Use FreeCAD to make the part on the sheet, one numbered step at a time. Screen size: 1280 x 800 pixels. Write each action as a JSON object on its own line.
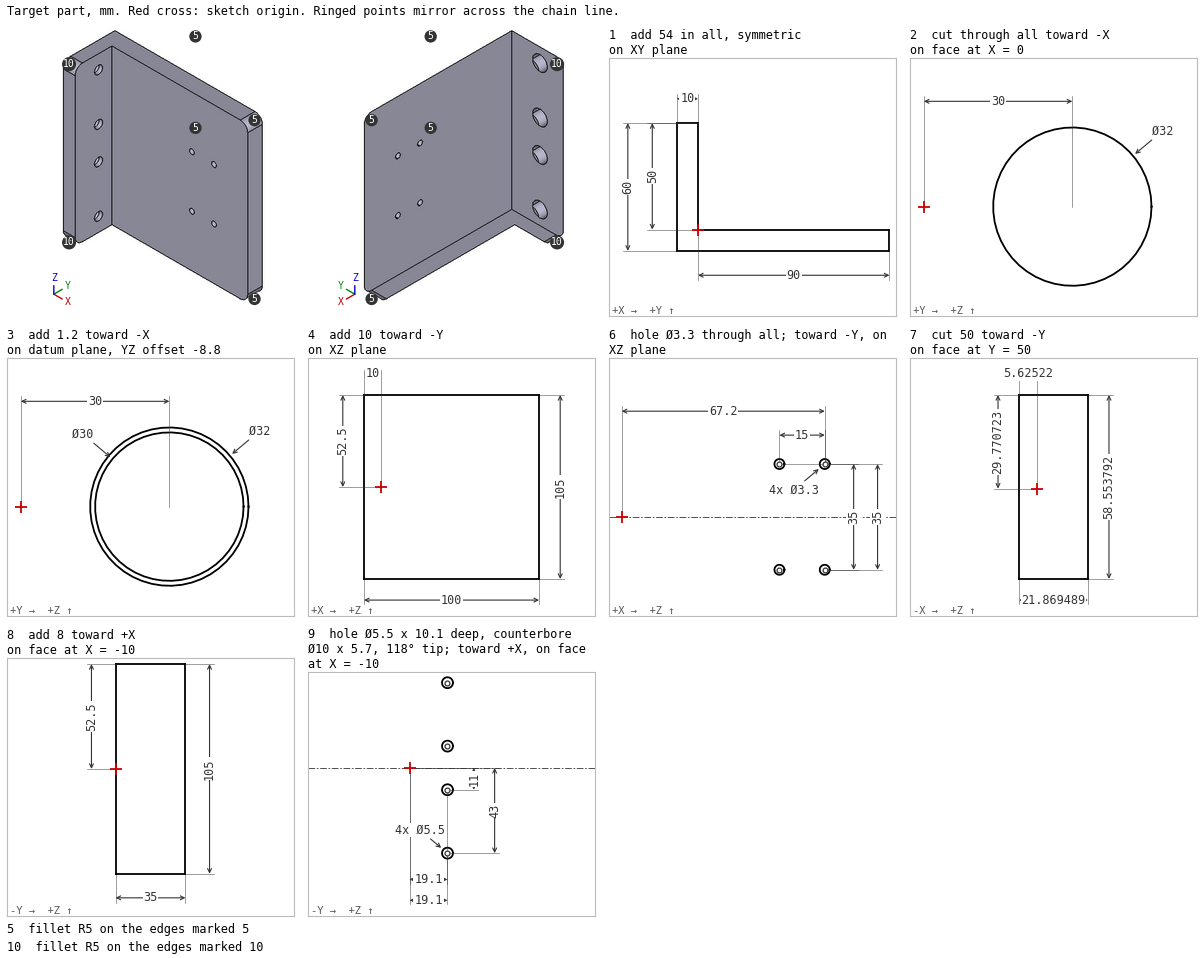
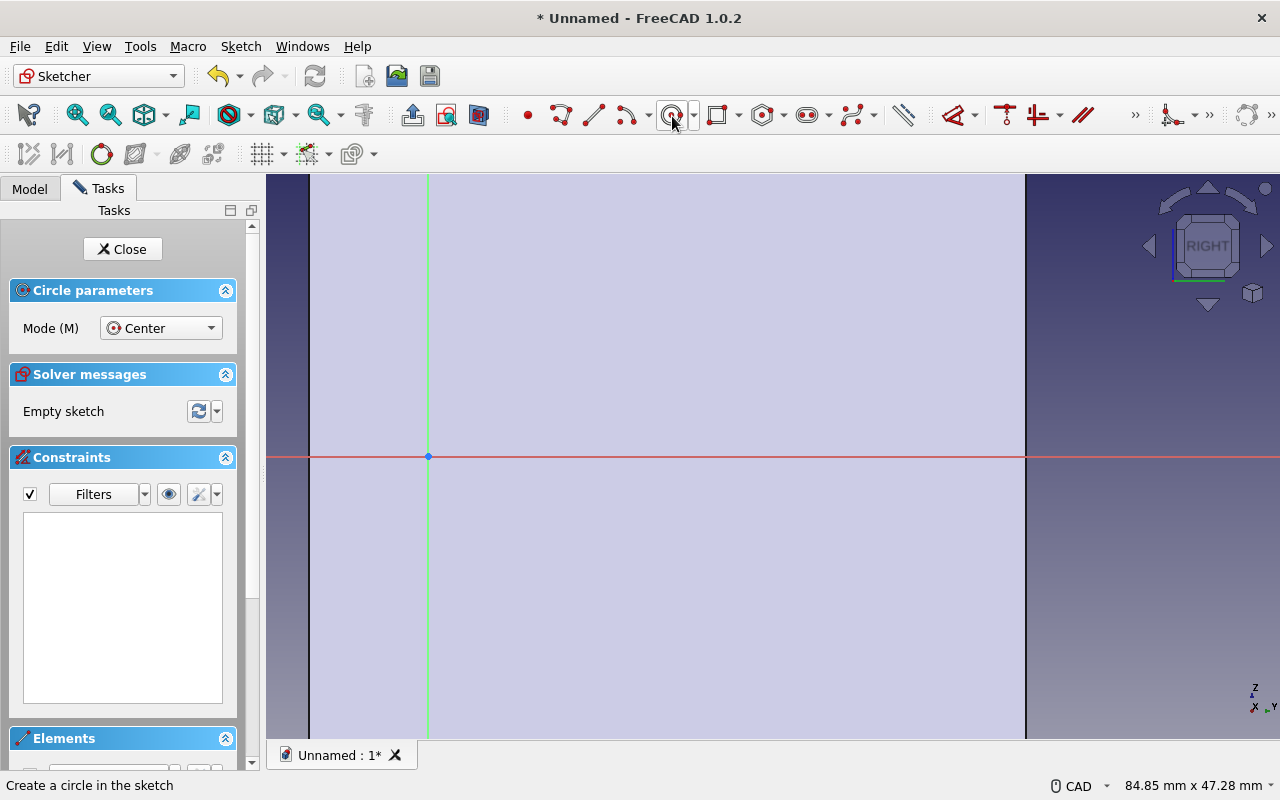
{"action": "left_click", "coordinate": [787, 456]}
{"action": "mouse_move", "coordinate": [922, 321]}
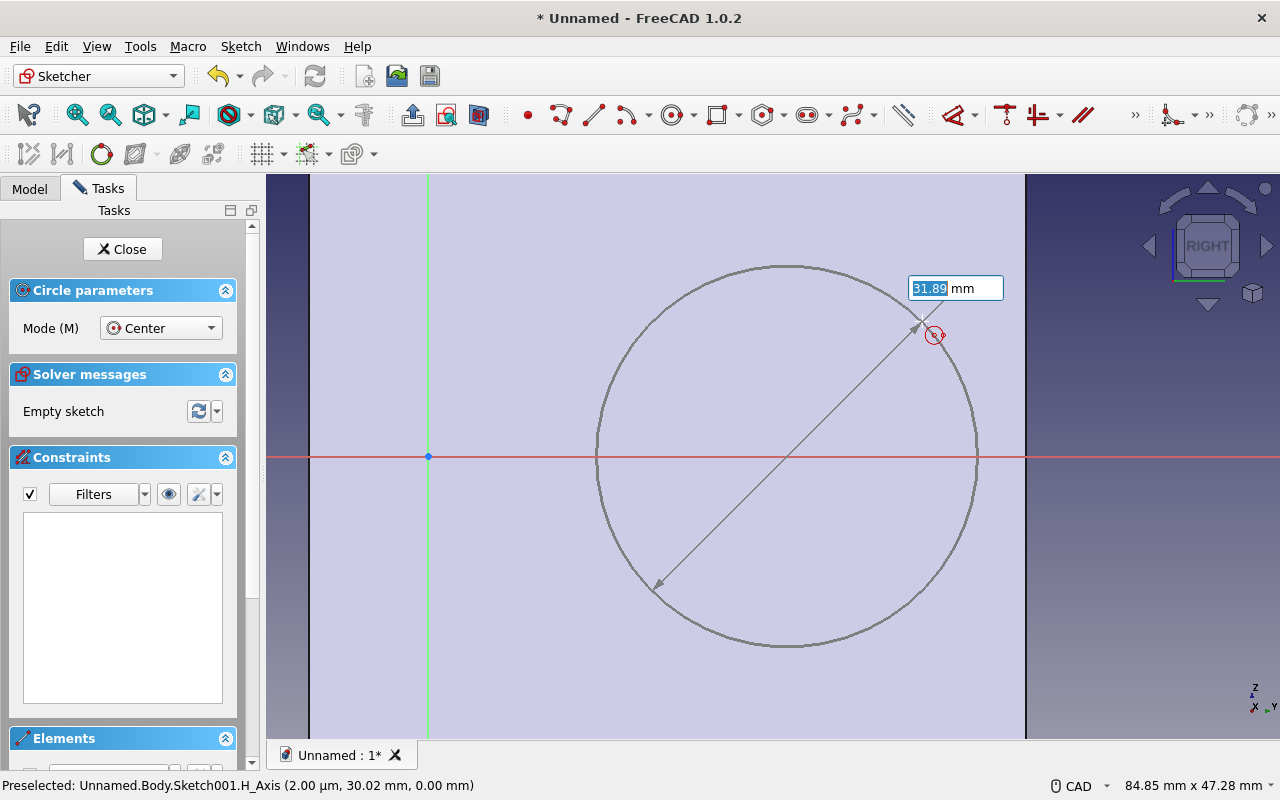
{"action": "type", "text": "32"}
{"action": "key", "text": "Return"}
{"action": "key", "text": "Escape"}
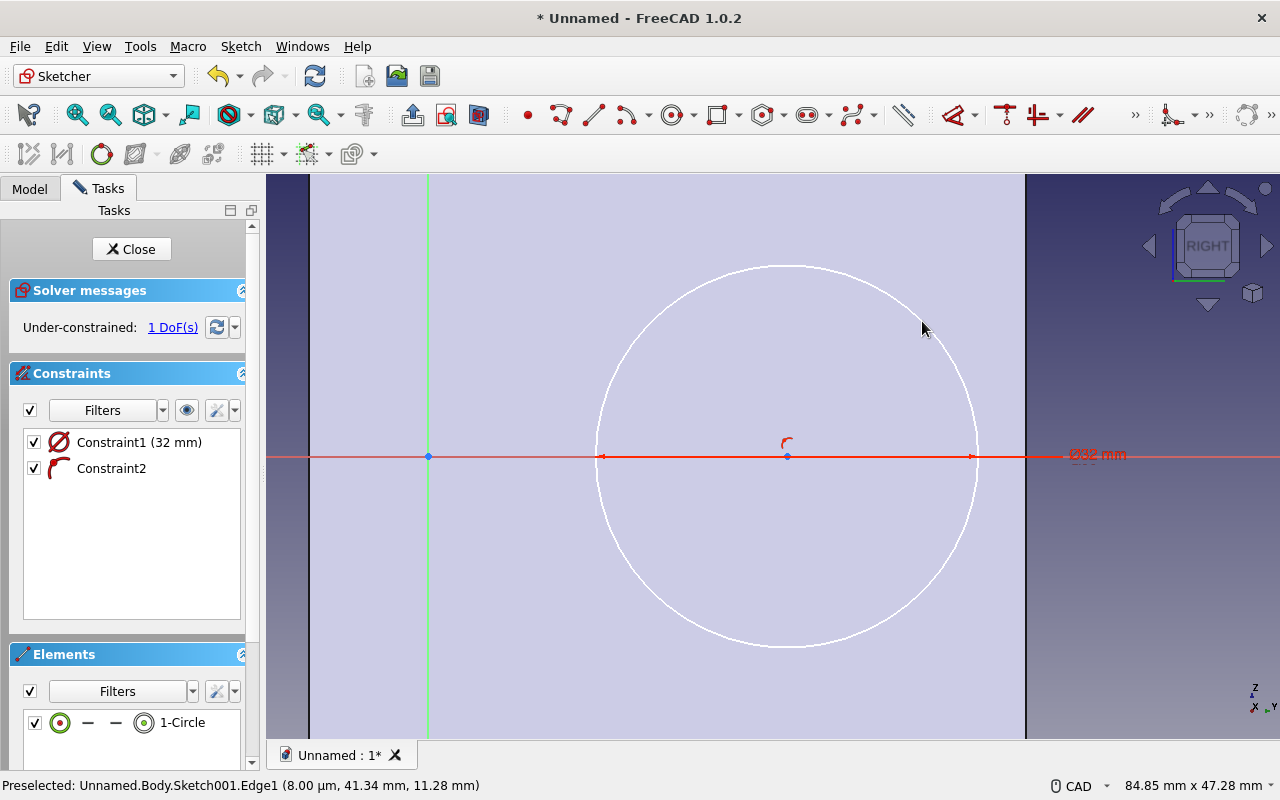
{"action": "left_click", "coordinate": [952, 116]}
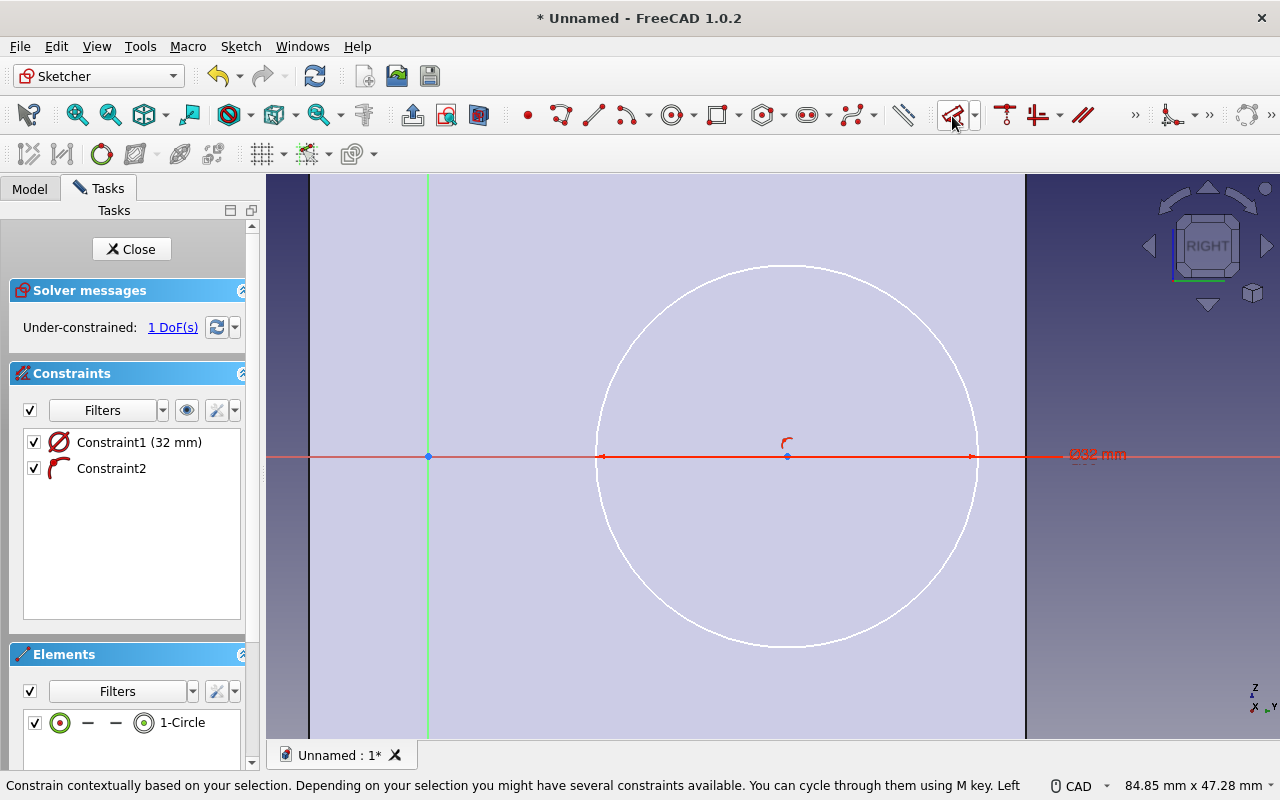
{"action": "left_click", "coordinate": [787, 456]}
{"action": "left_click", "coordinate": [525, 490]}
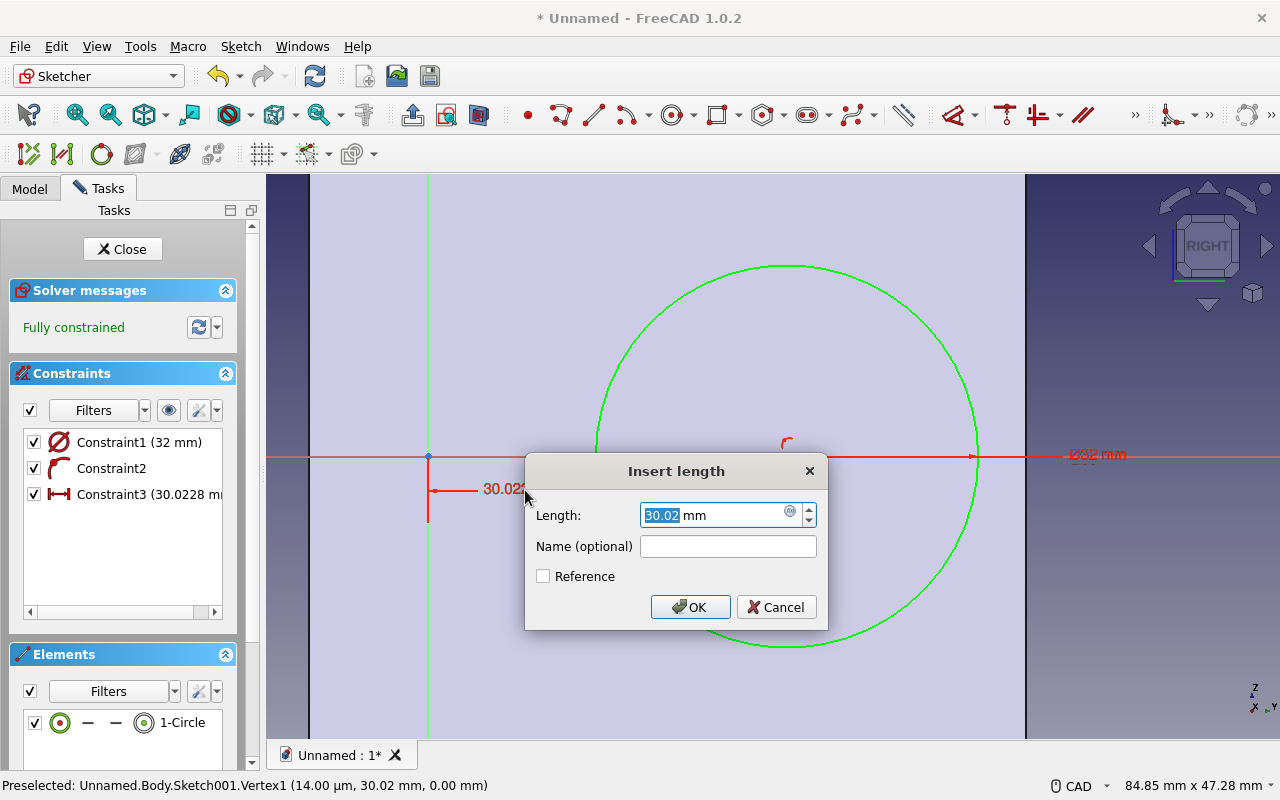
{"action": "type", "text": "30"}
{"action": "key", "text": "Return"}
{"action": "key", "text": "Escape"}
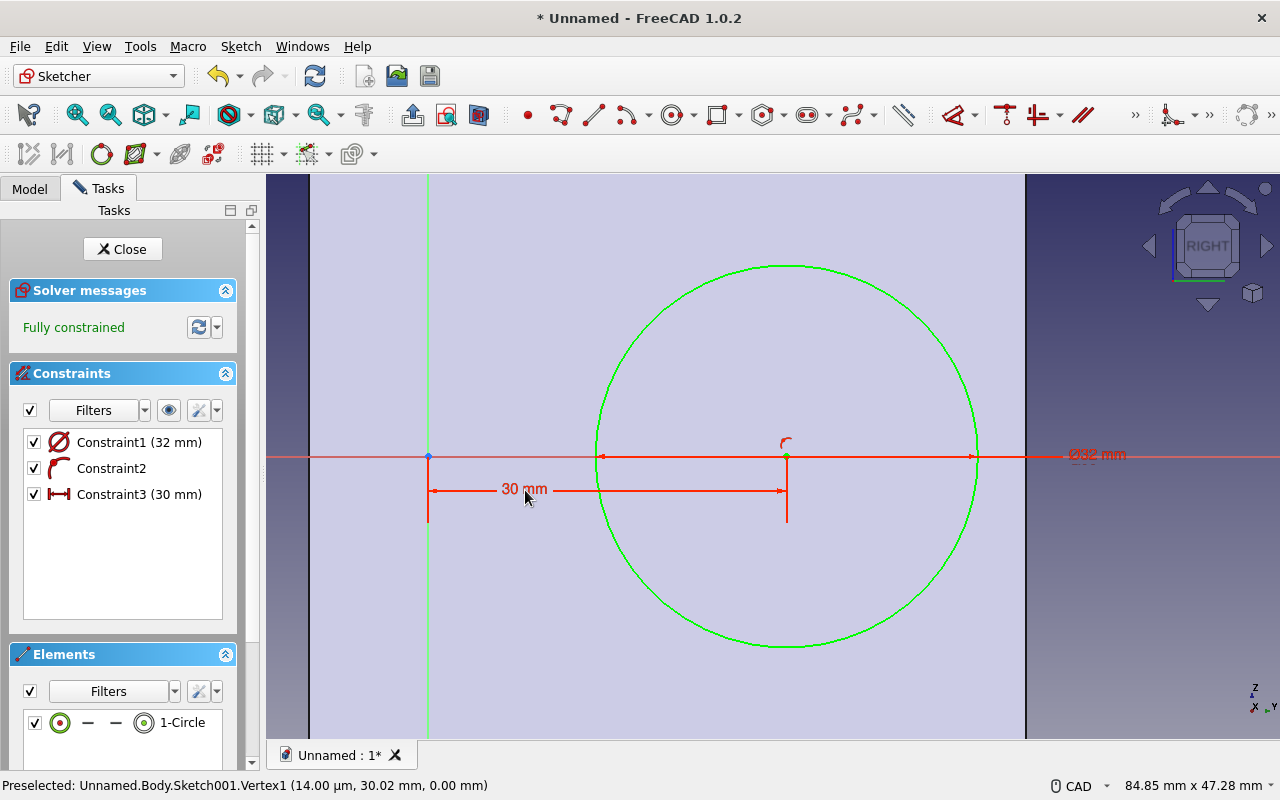
{"action": "left_click", "coordinate": [123, 249]}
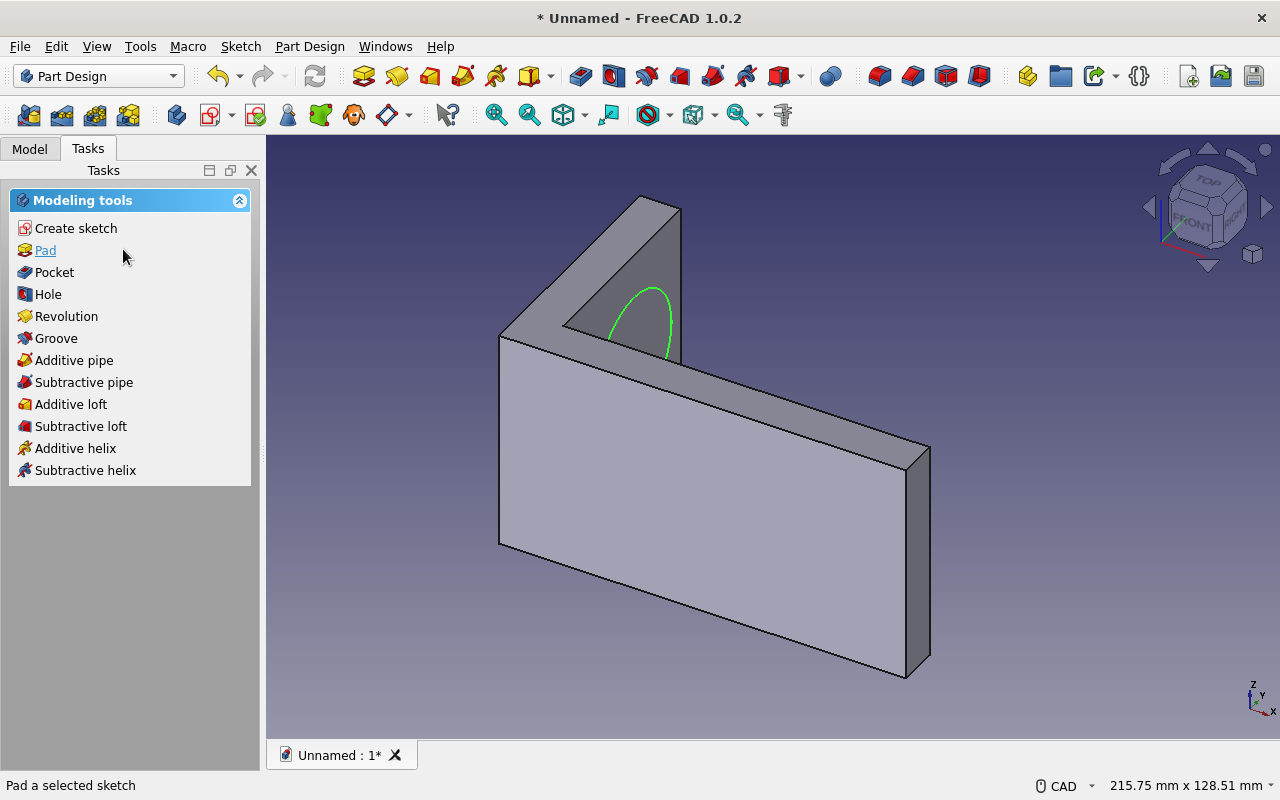
{"action": "left_click", "coordinate": [581, 76]}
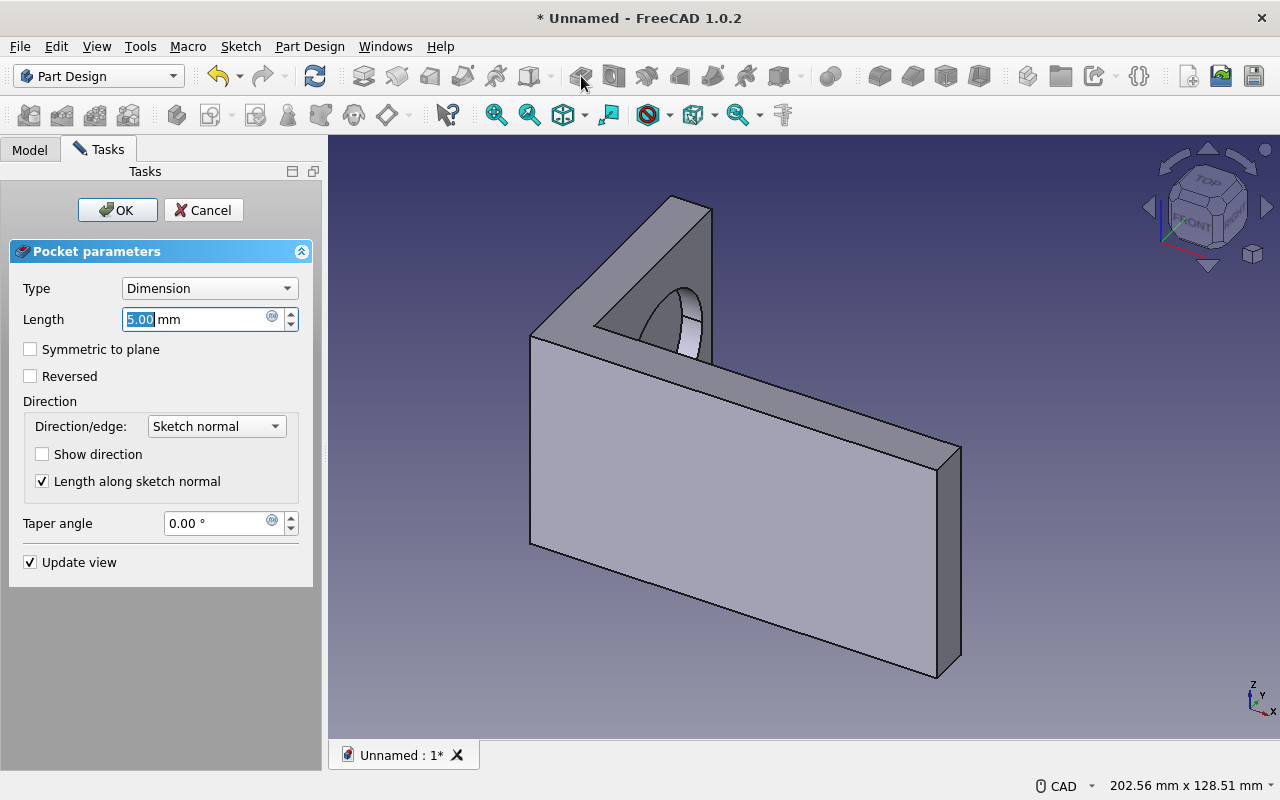
{"action": "left_click", "coordinate": [210, 288]}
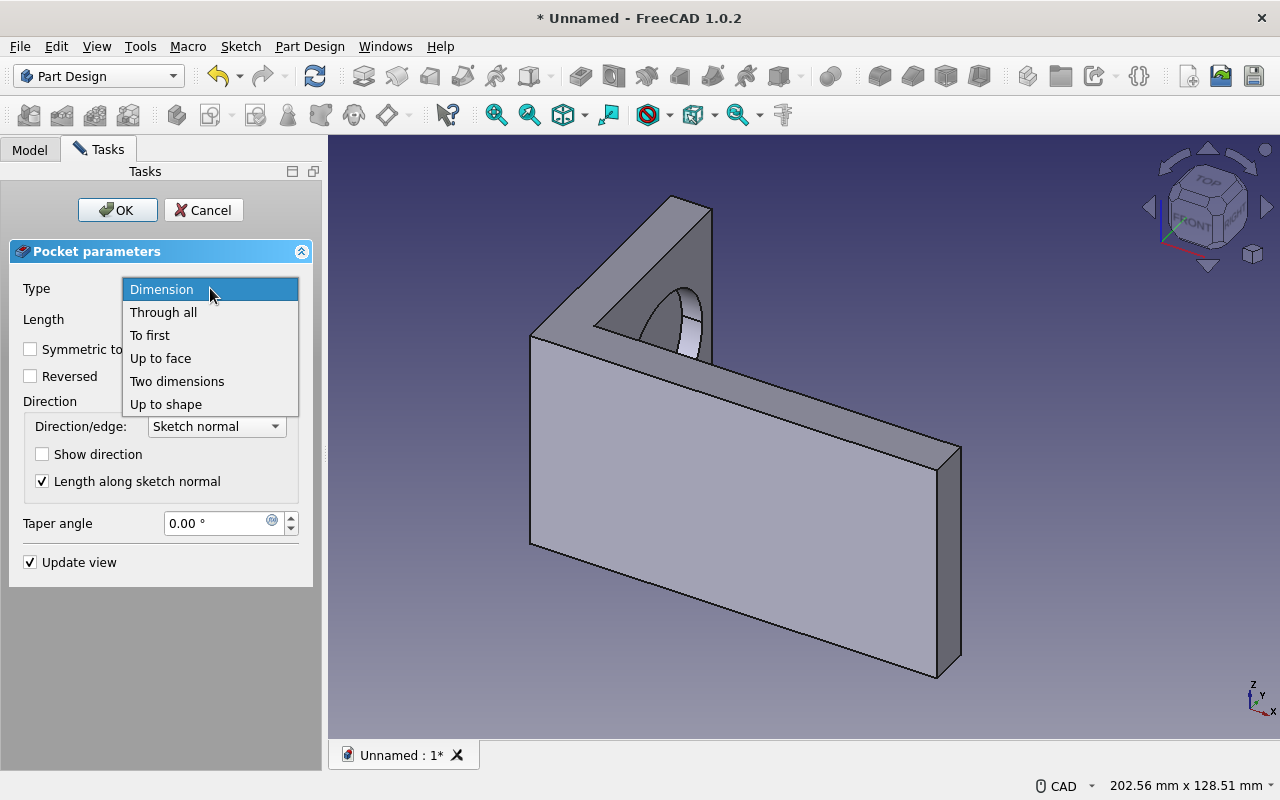
{"action": "left_click", "coordinate": [208, 312]}